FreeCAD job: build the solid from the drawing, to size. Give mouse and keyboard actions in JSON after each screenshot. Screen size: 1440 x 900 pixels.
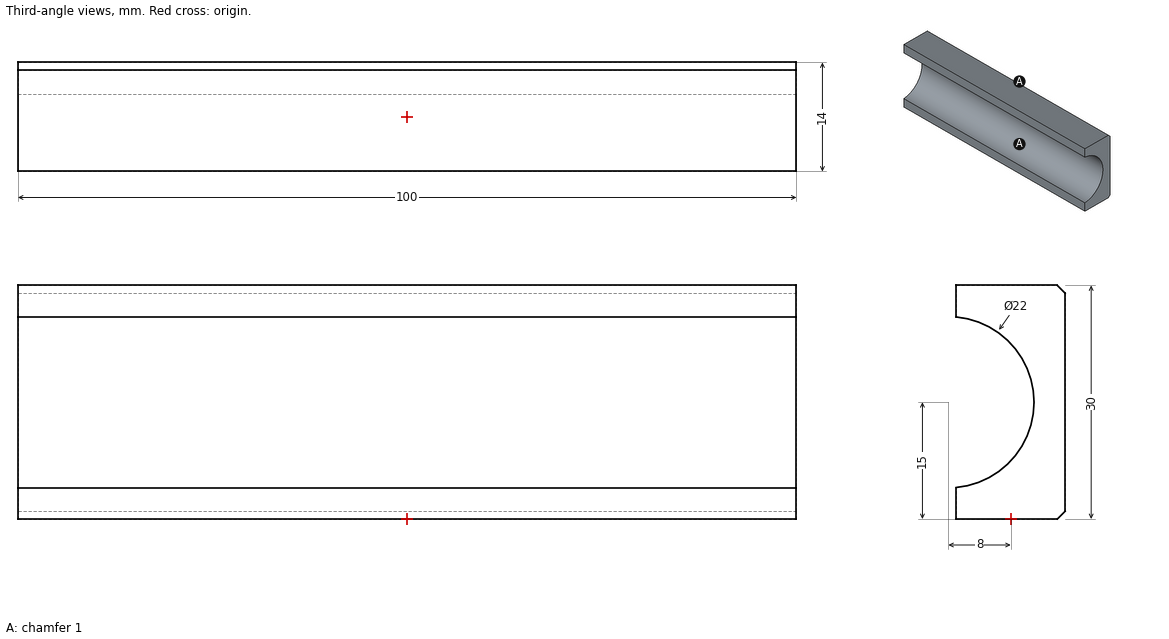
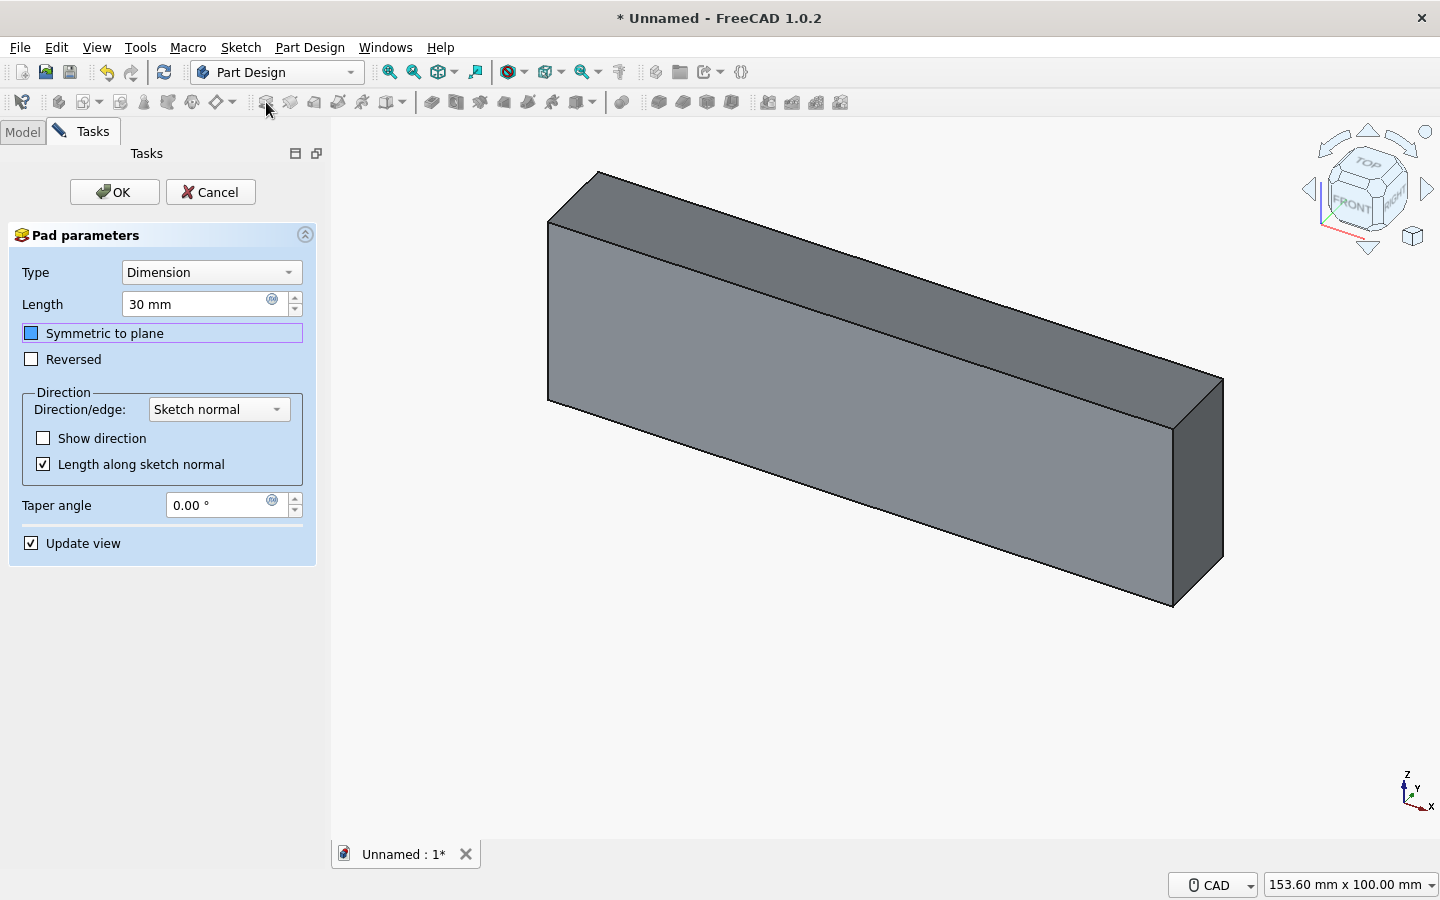
{"action": "left_click", "coordinate": [115, 192]}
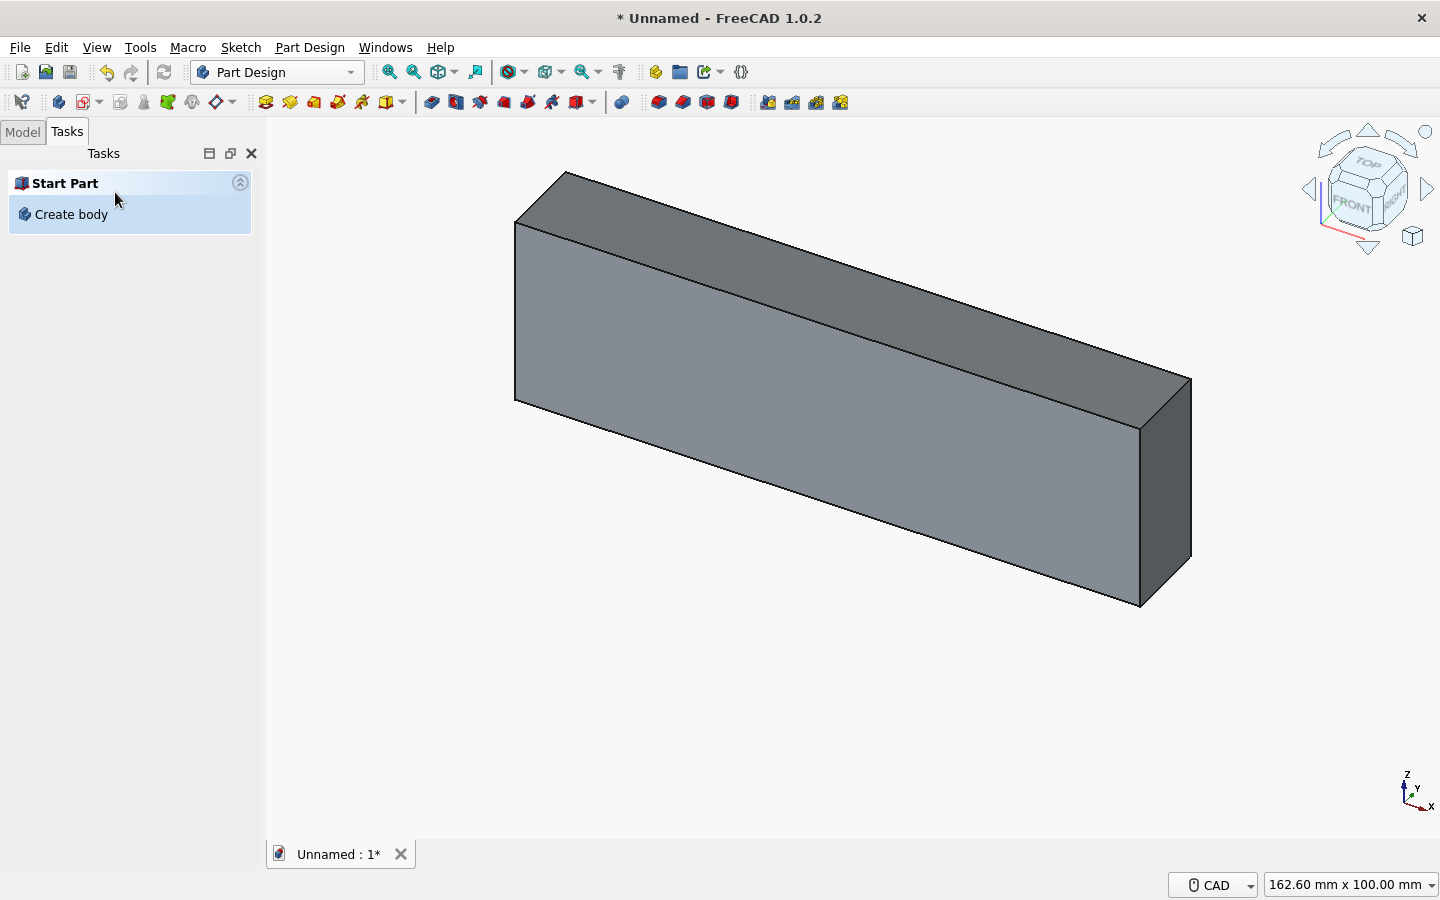
{"action": "key", "text": "6"}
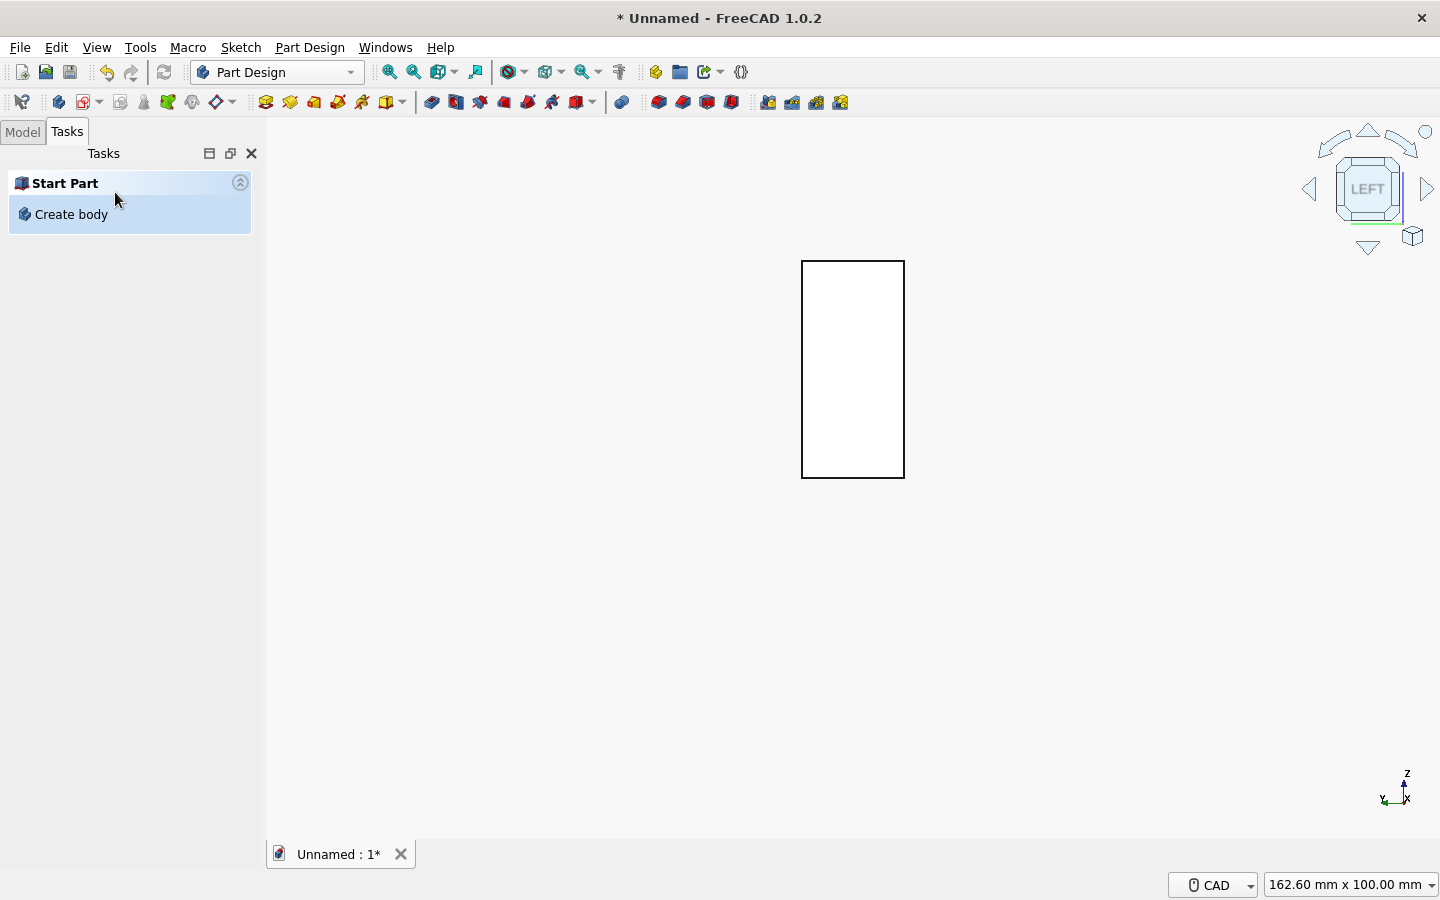
{"action": "key", "text": "v f"}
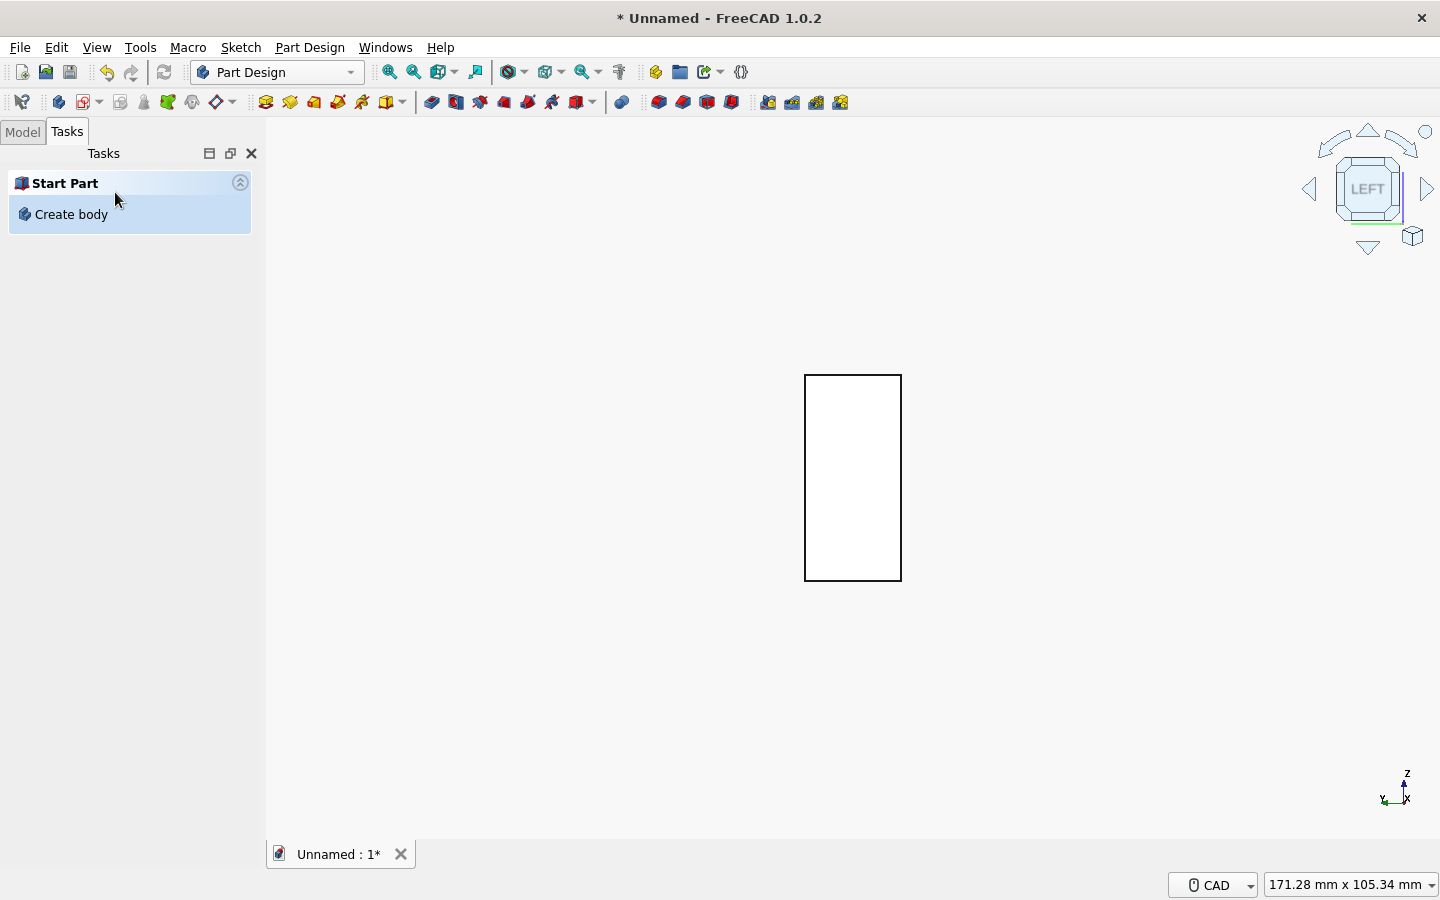
{"action": "left_click", "coordinate": [853, 448]}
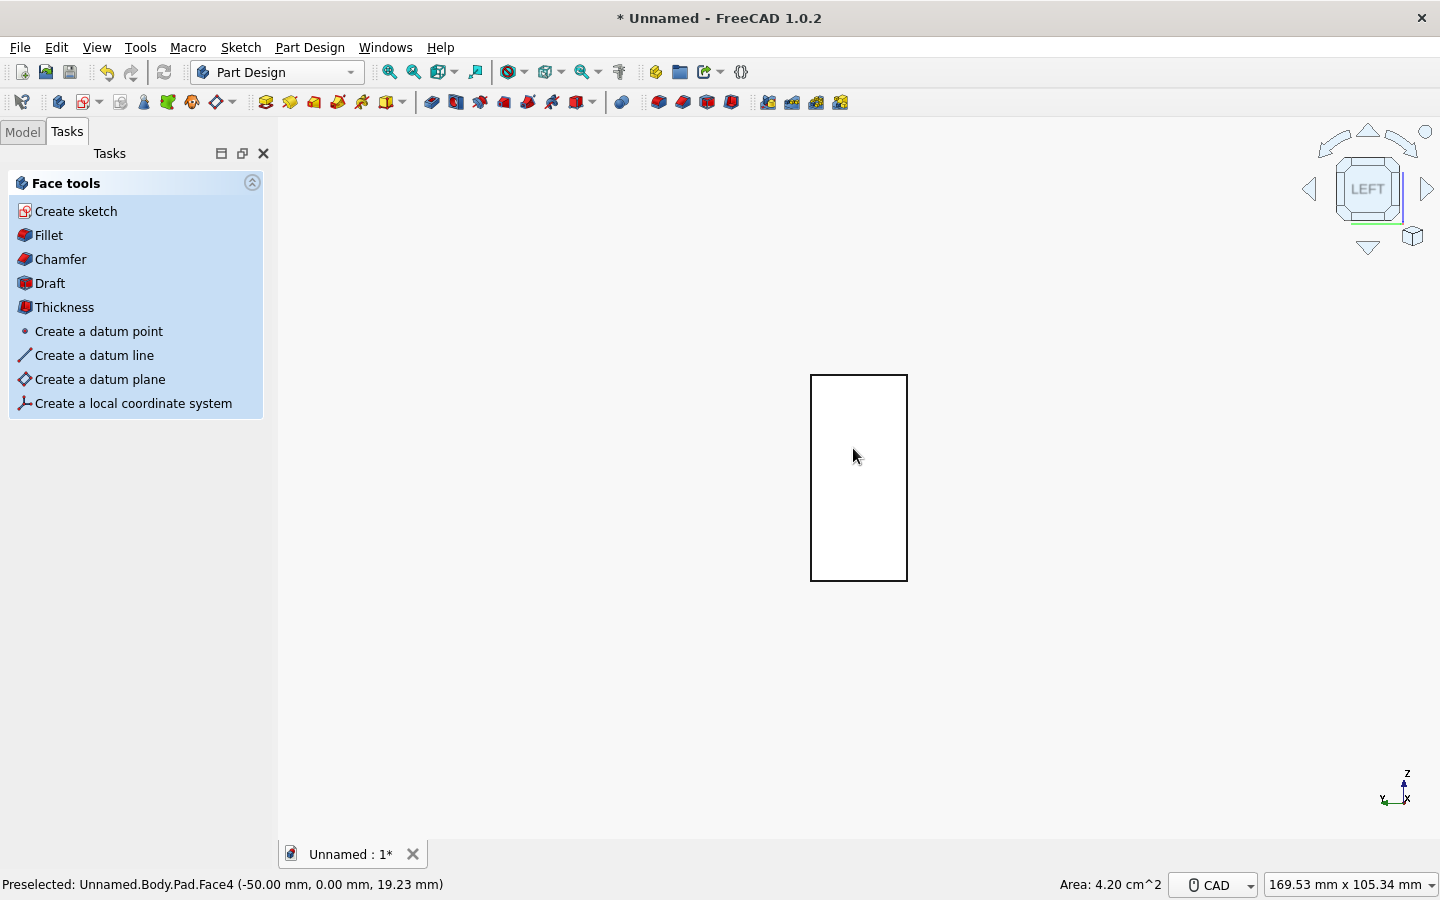
{"action": "left_click", "coordinate": [84, 102]}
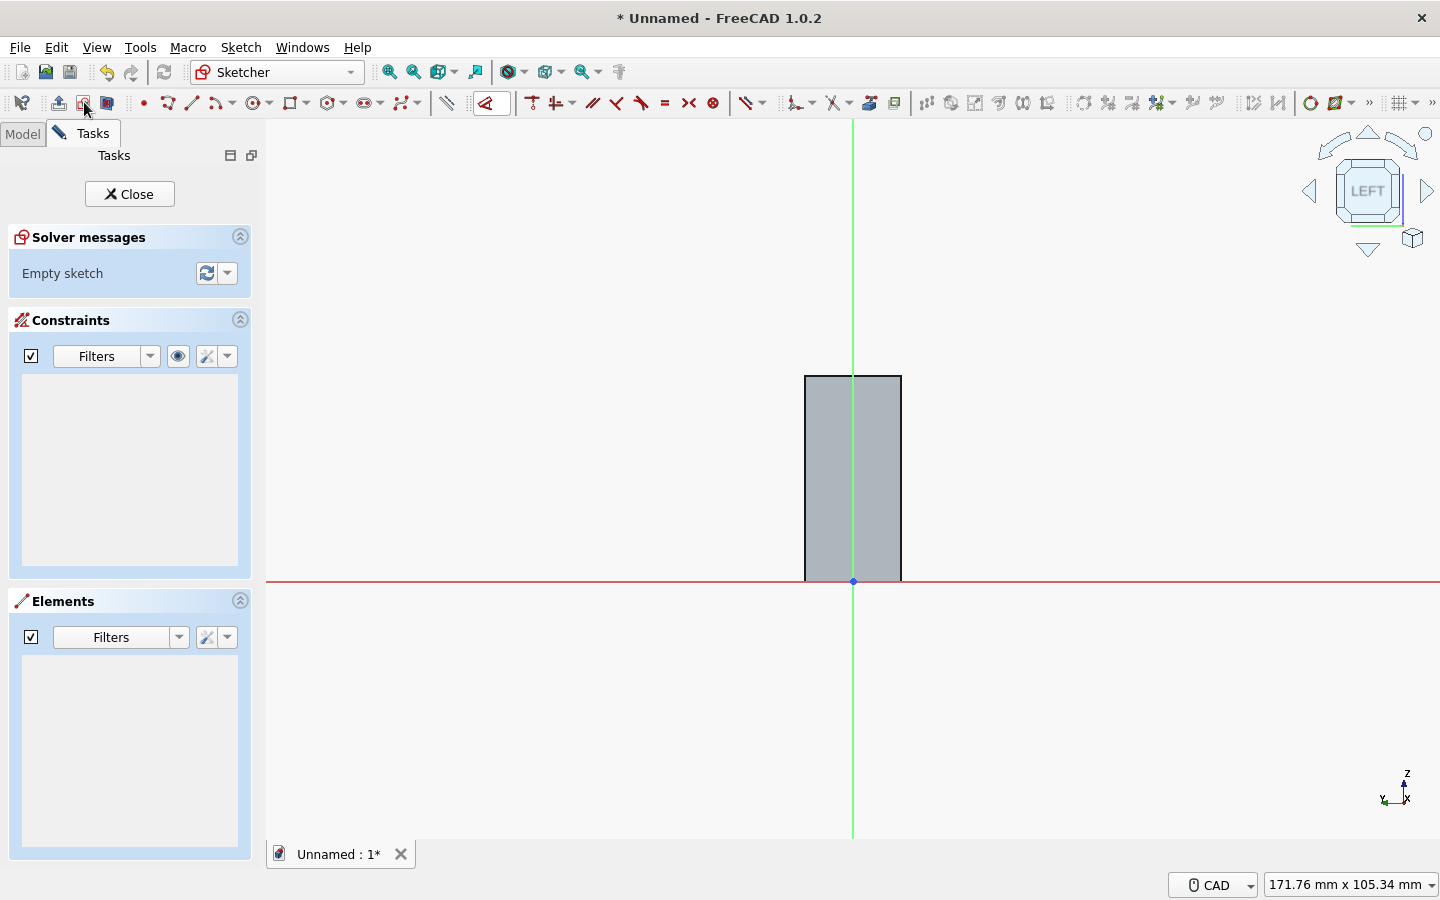
{"action": "scroll", "coordinate": [979, 501], "scroll_direction": "up", "scroll_amount": 5}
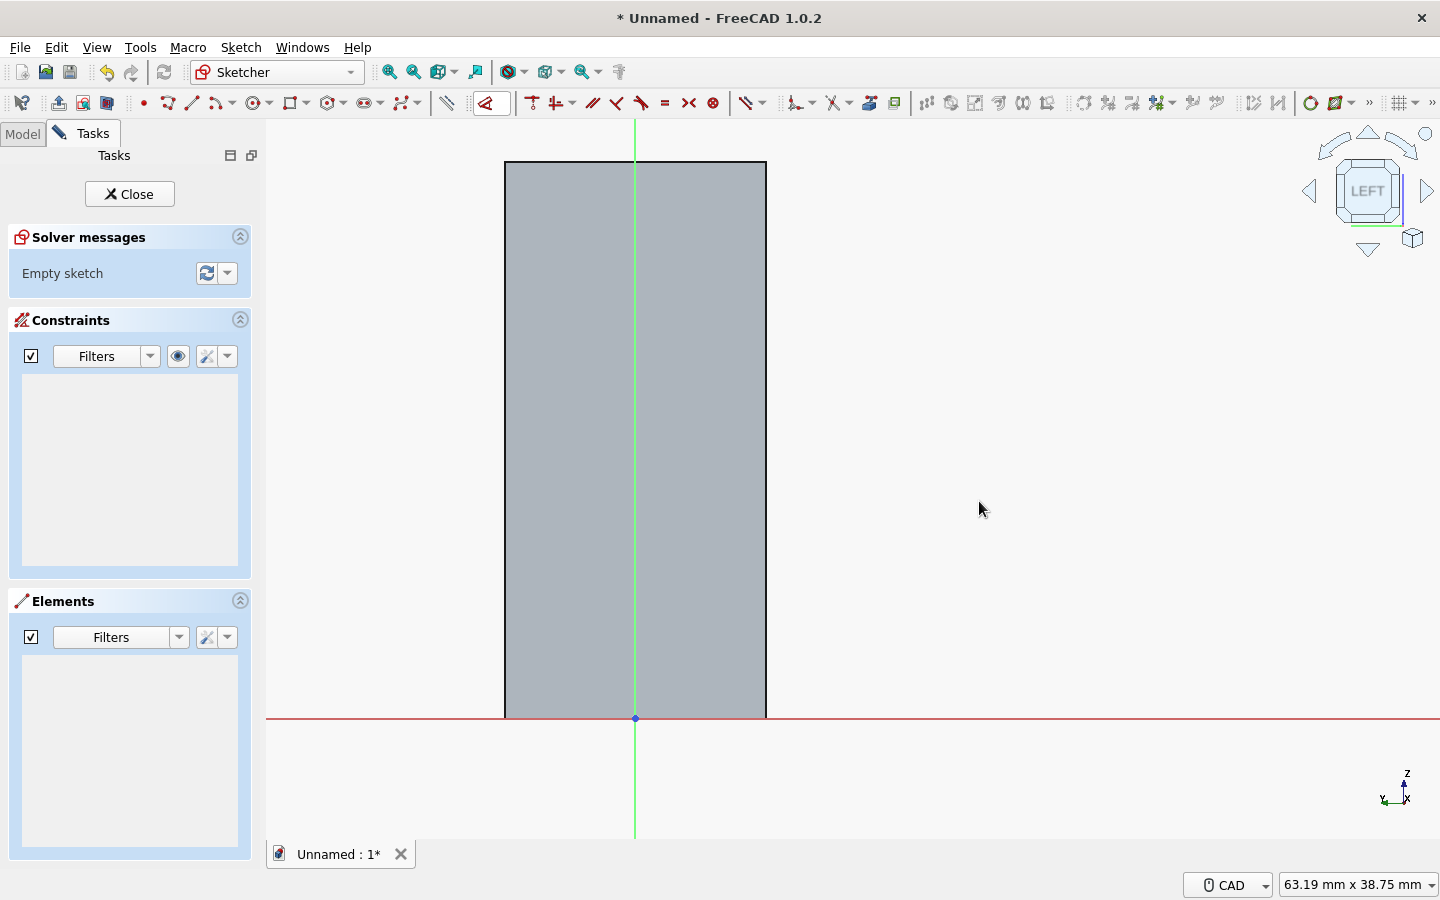
{"action": "left_click", "coordinate": [254, 104]}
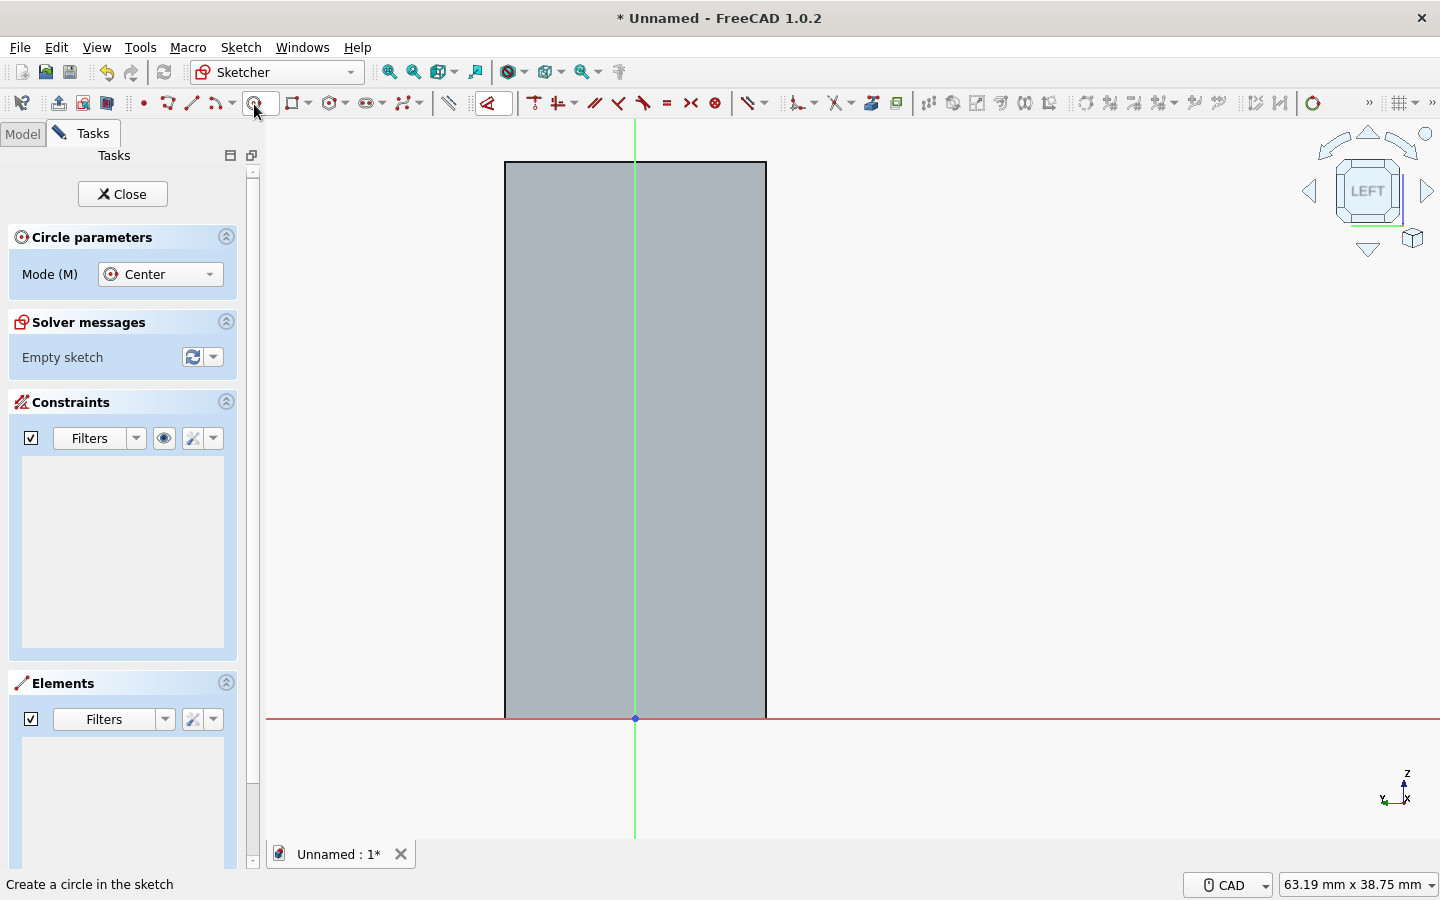
{"action": "left_click", "coordinate": [784, 440]}
{"action": "left_click", "coordinate": [929, 296]}
{"action": "key", "text": "Escape"}